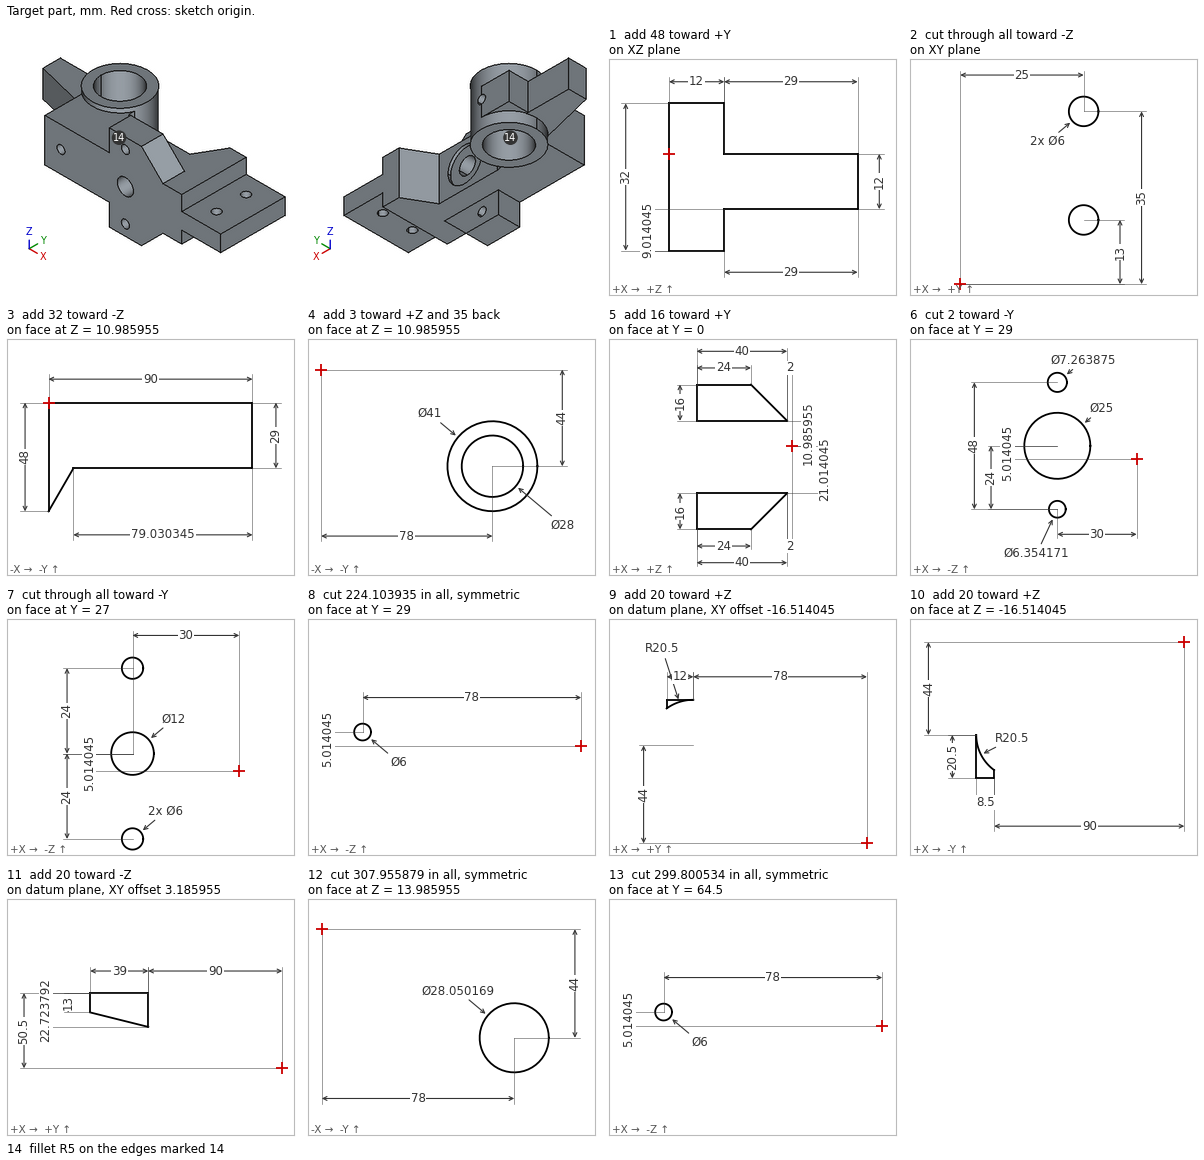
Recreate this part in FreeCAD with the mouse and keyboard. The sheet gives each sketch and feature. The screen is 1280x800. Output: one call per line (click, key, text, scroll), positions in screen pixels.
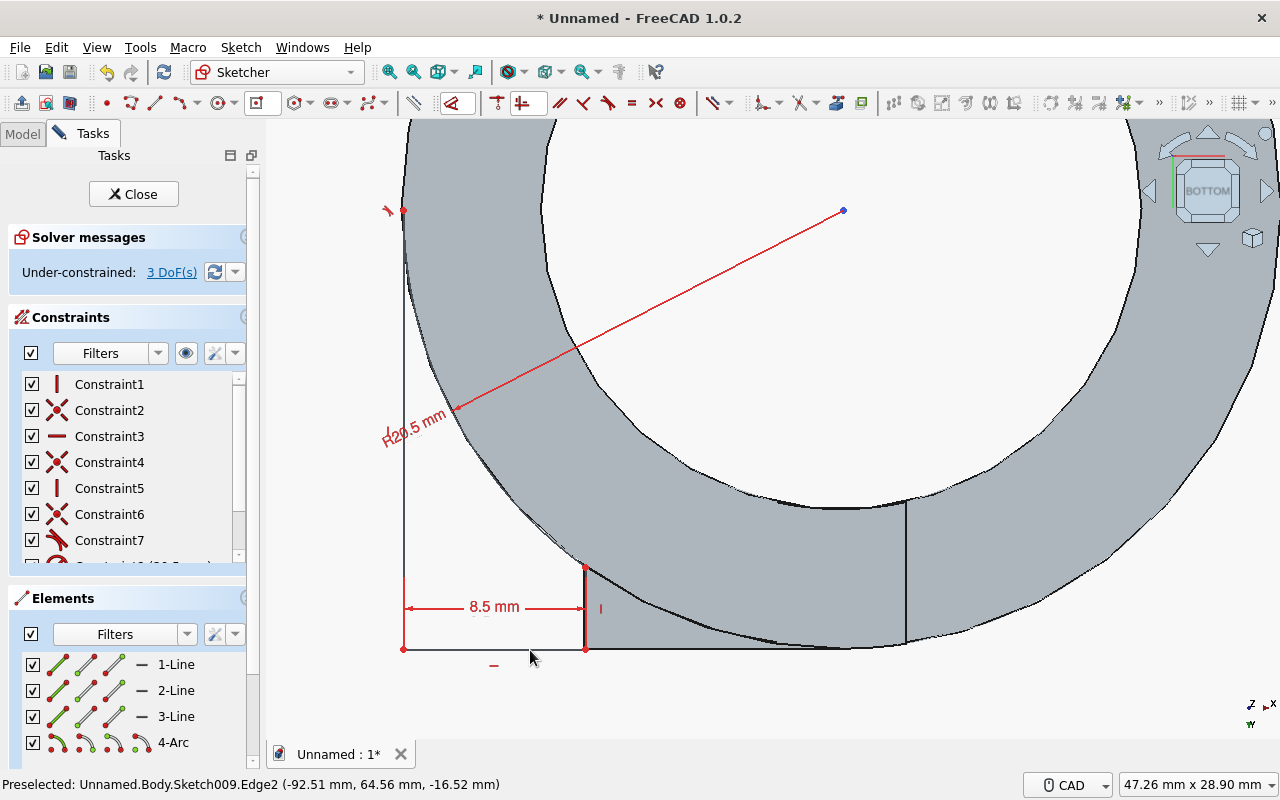
click(586, 567)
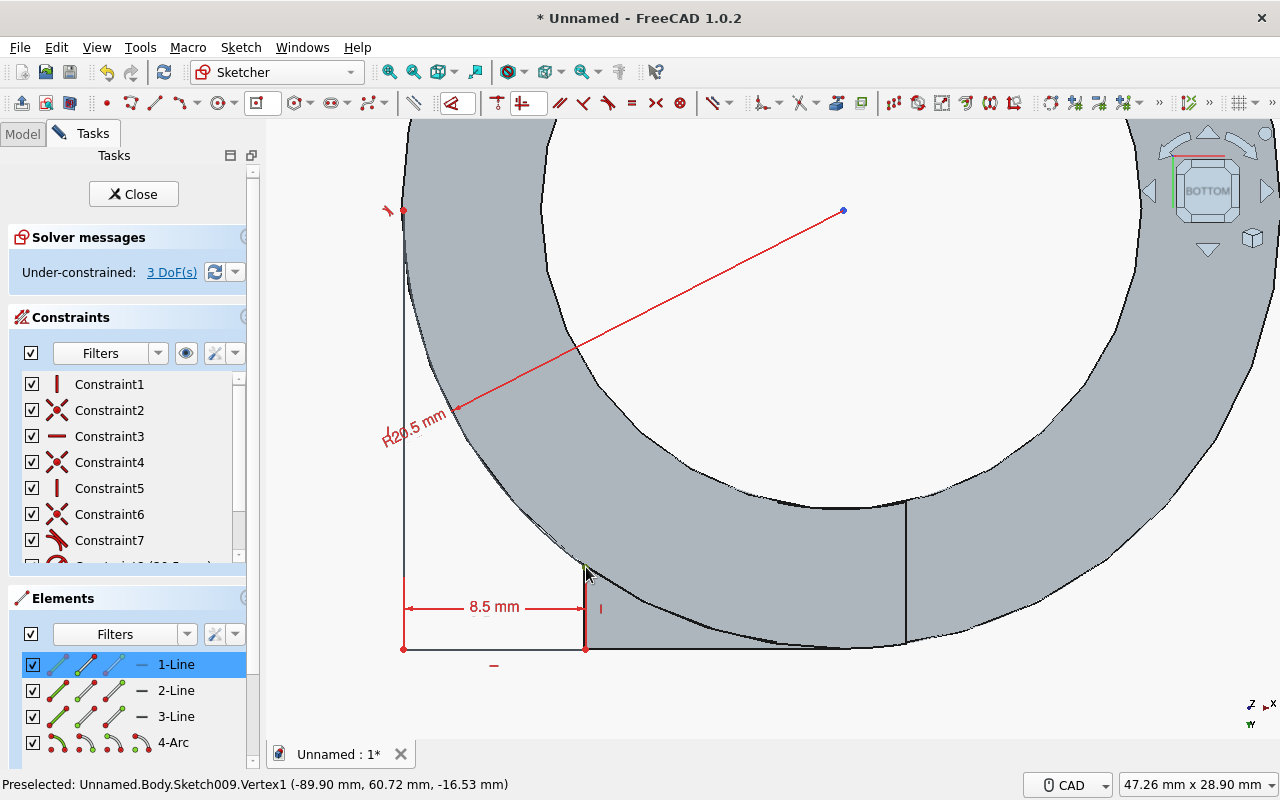
click(470, 104)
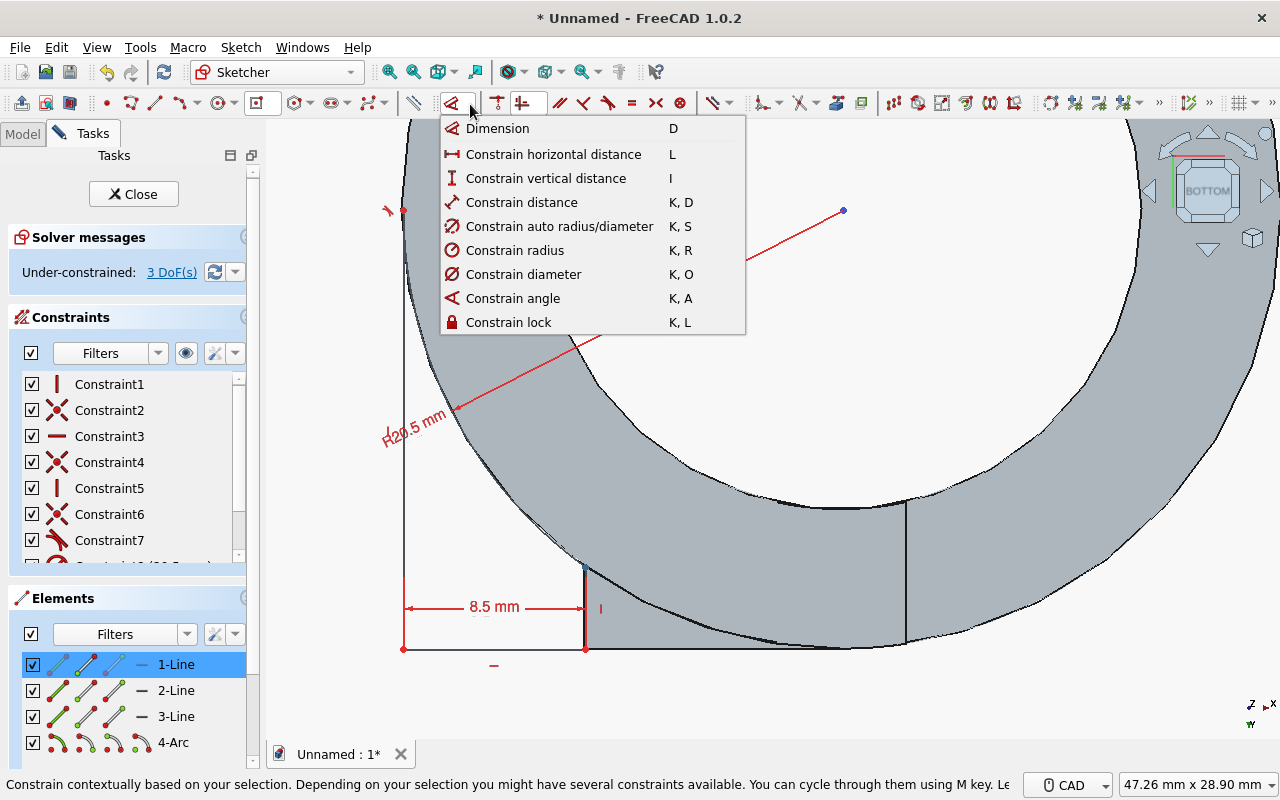
click(593, 154)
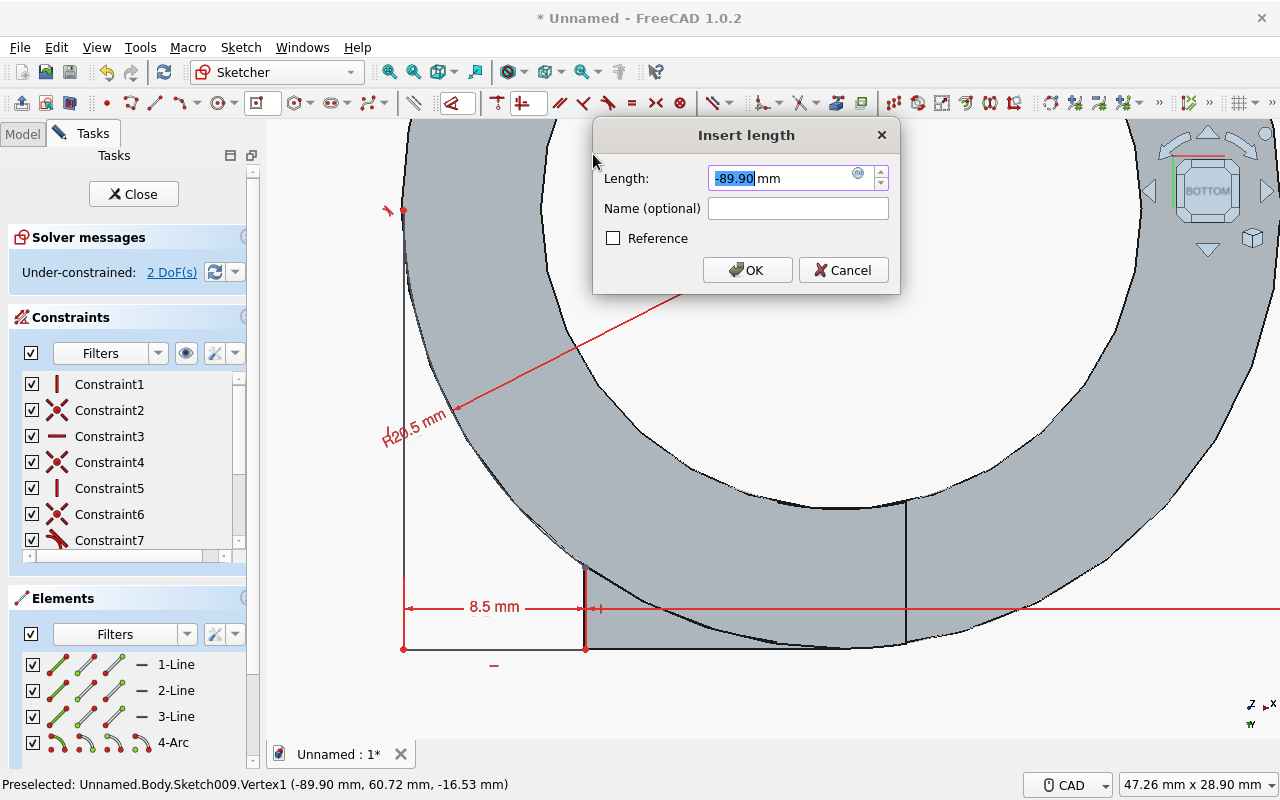
text(-90)
key(Return)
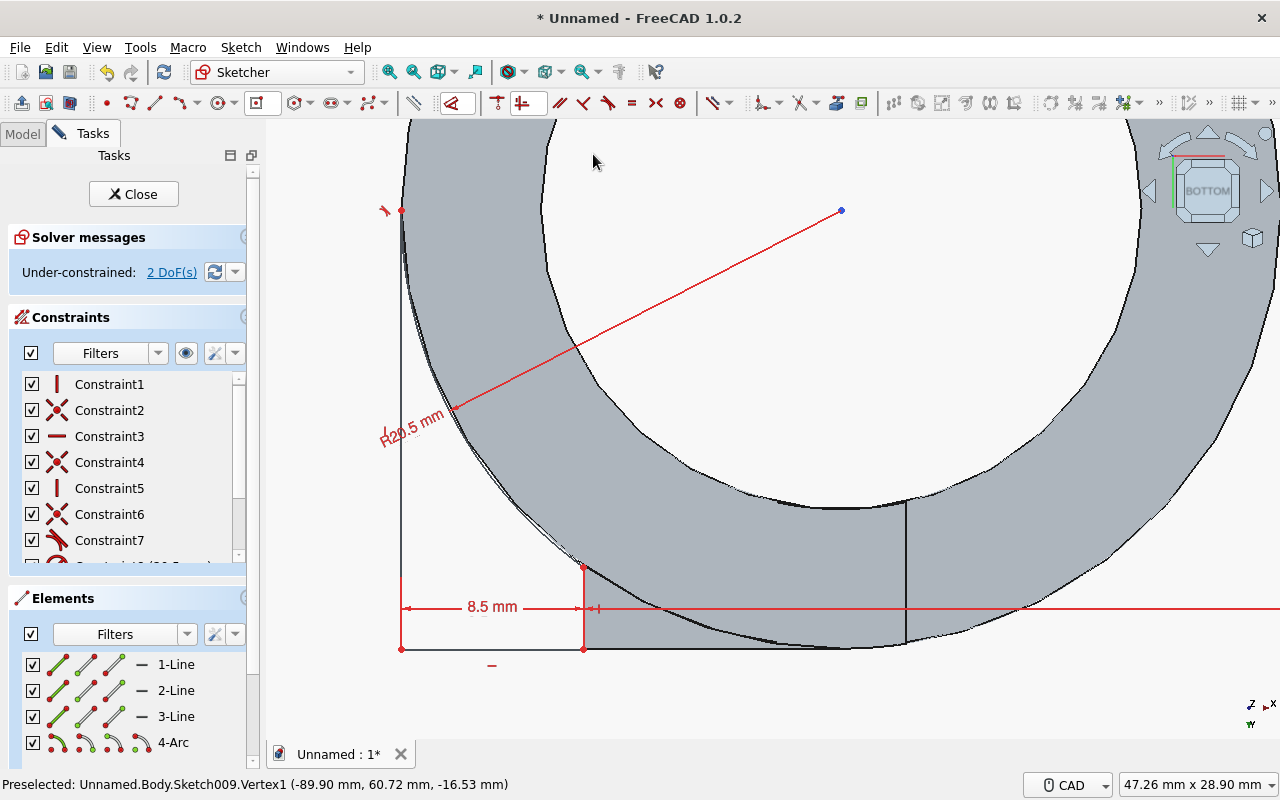
click(401, 211)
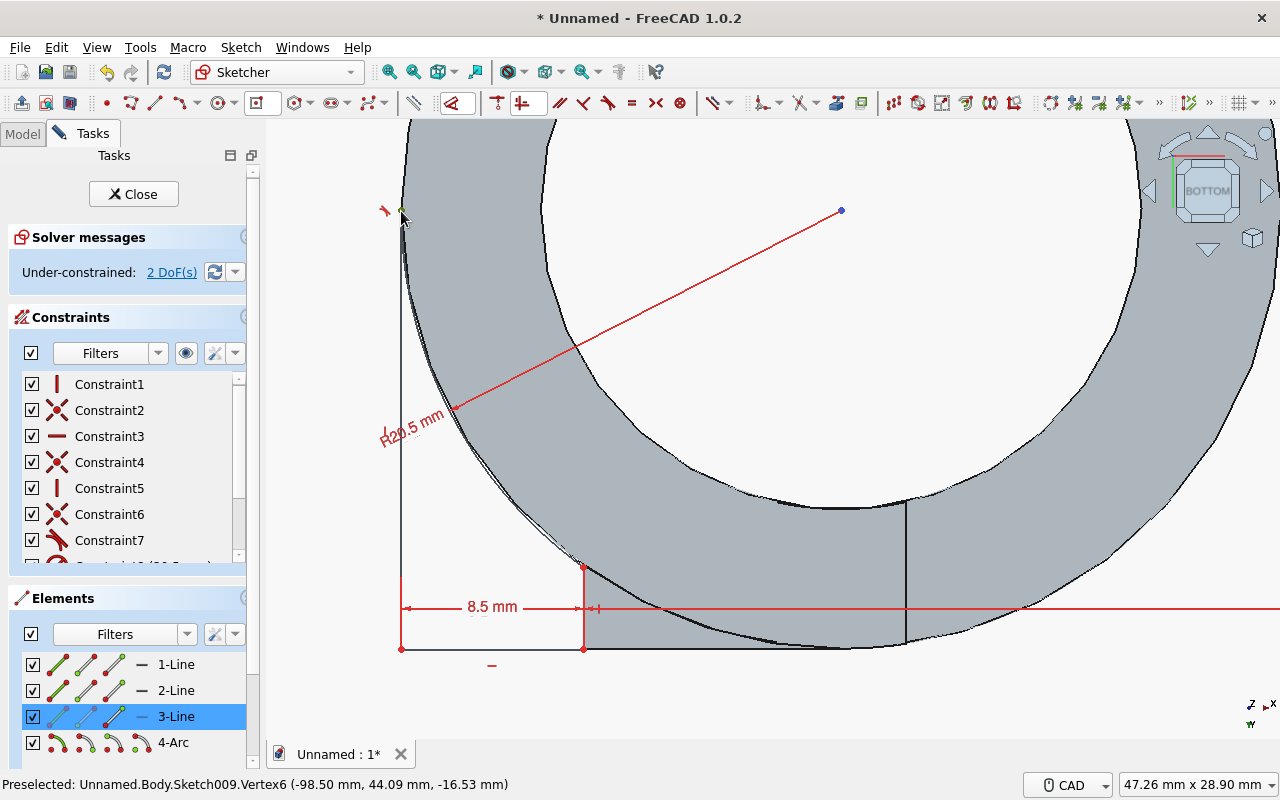
key(i)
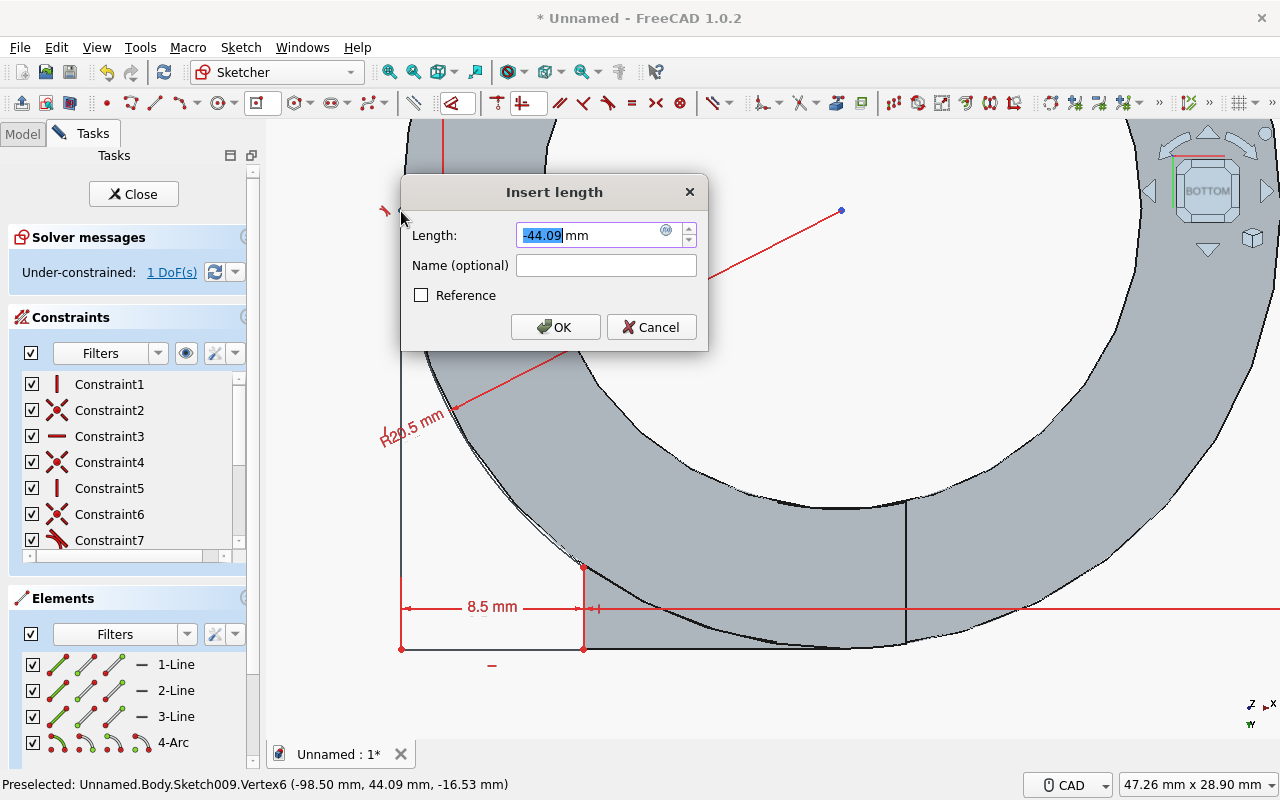
text(-44)
key(Return)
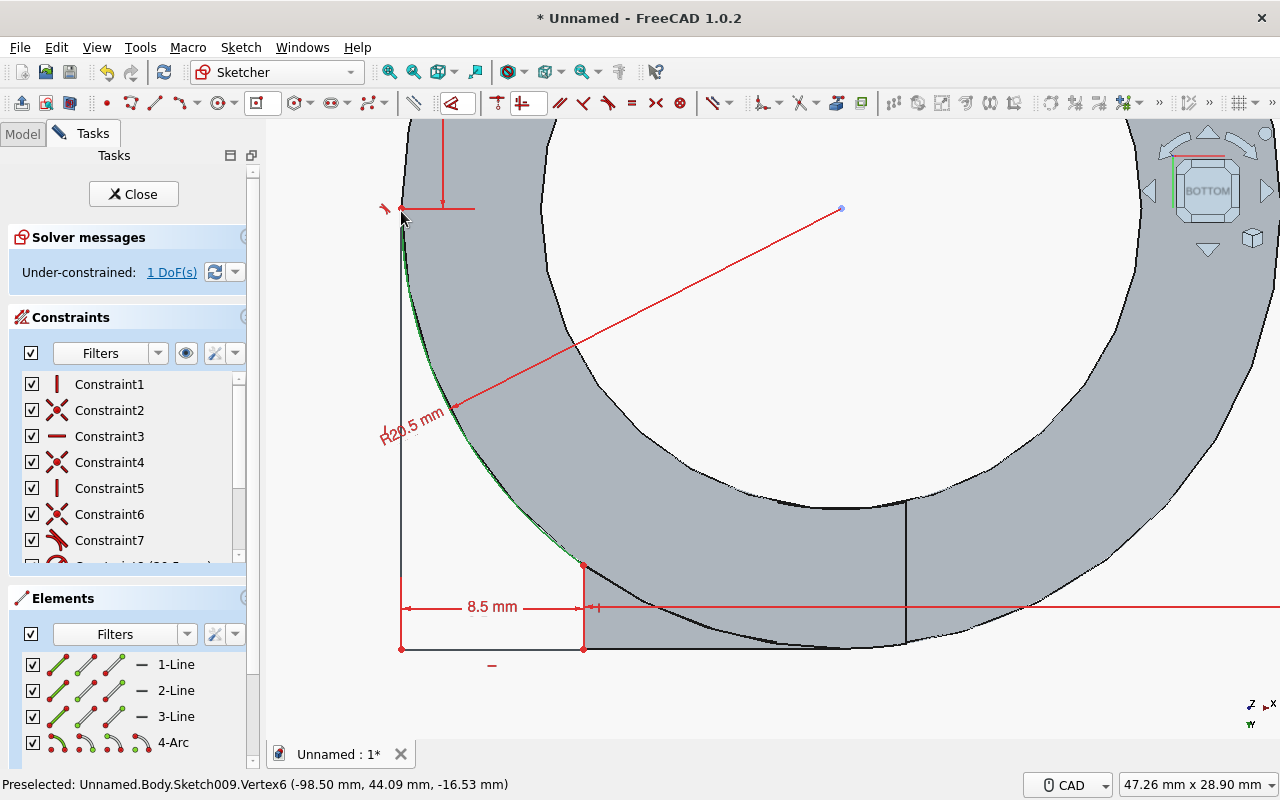
click(401, 518)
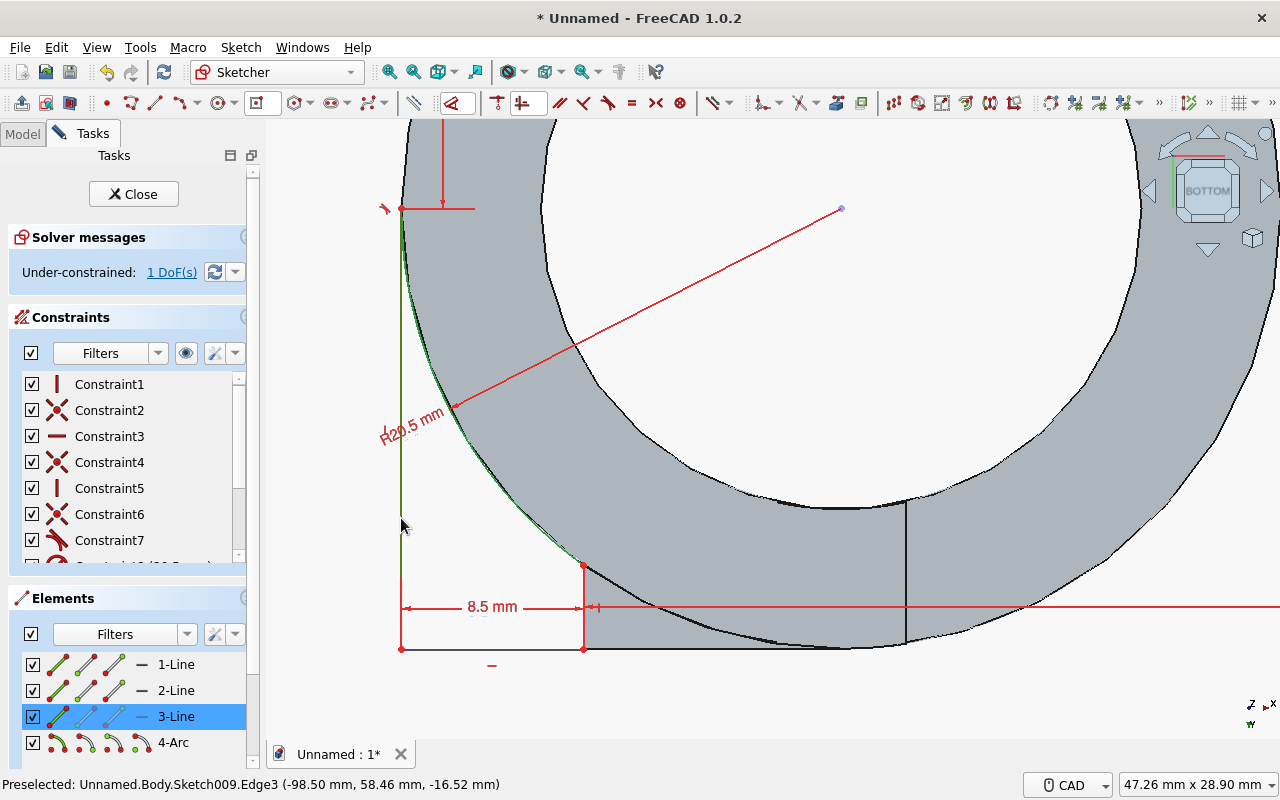
click(470, 104)